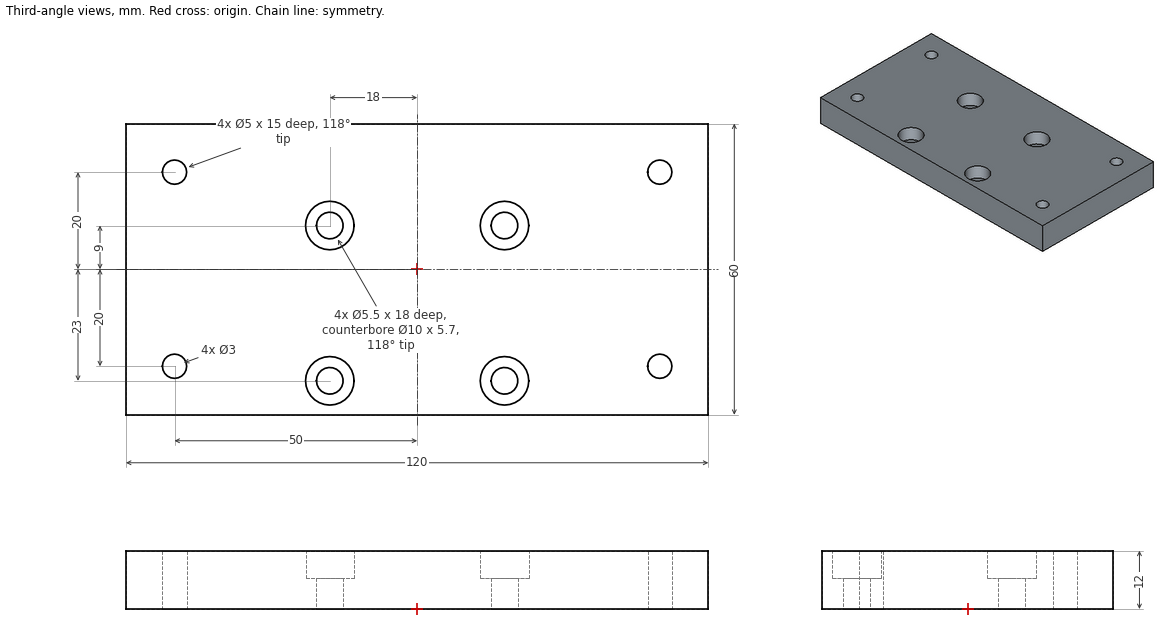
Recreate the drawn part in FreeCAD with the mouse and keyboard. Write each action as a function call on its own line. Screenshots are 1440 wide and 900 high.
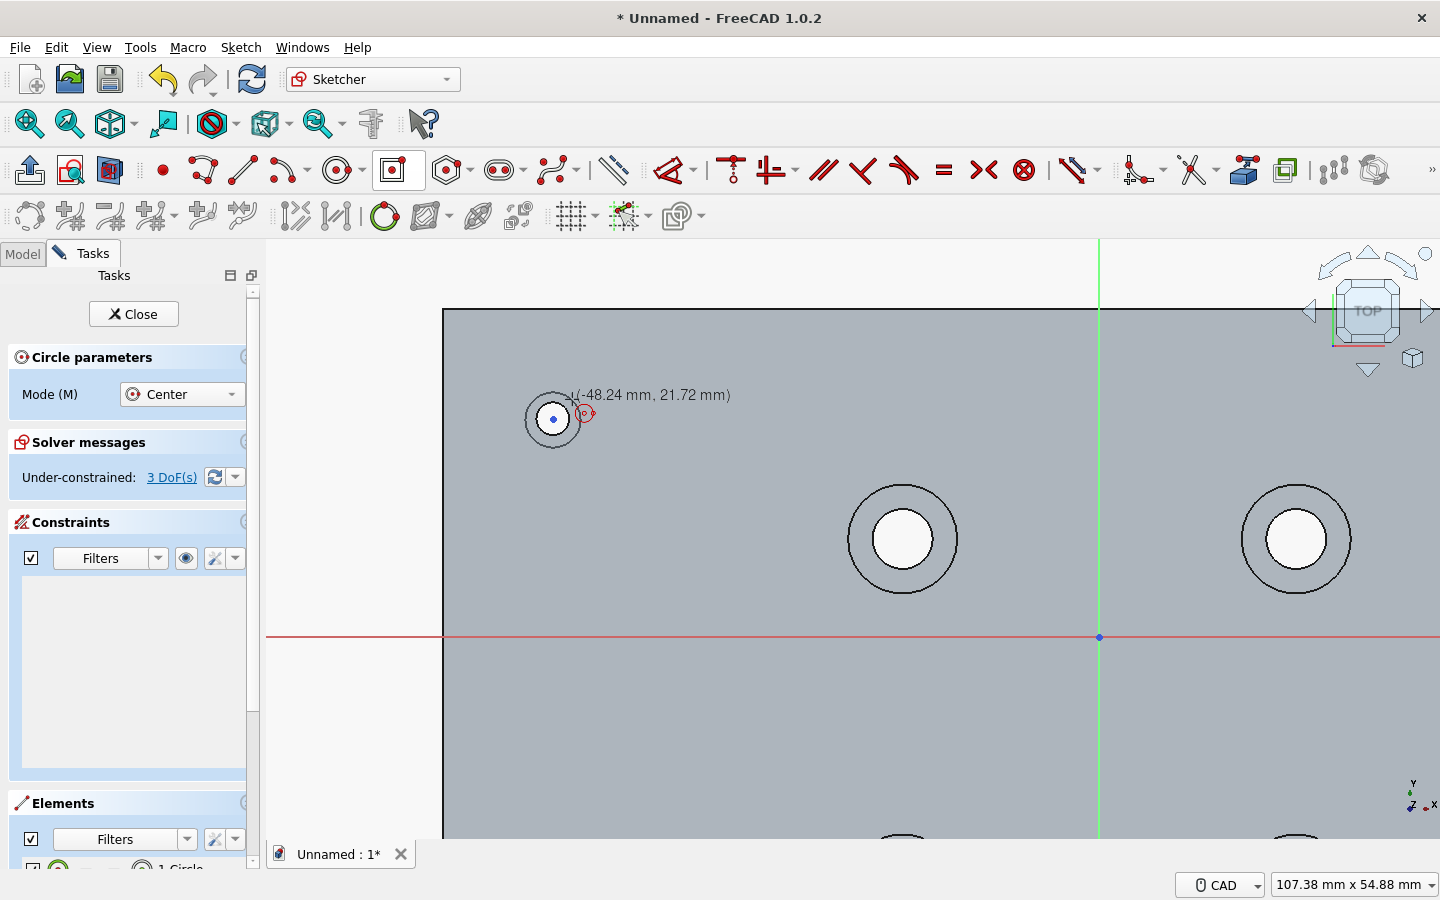
scroll(401, 419, down, 3)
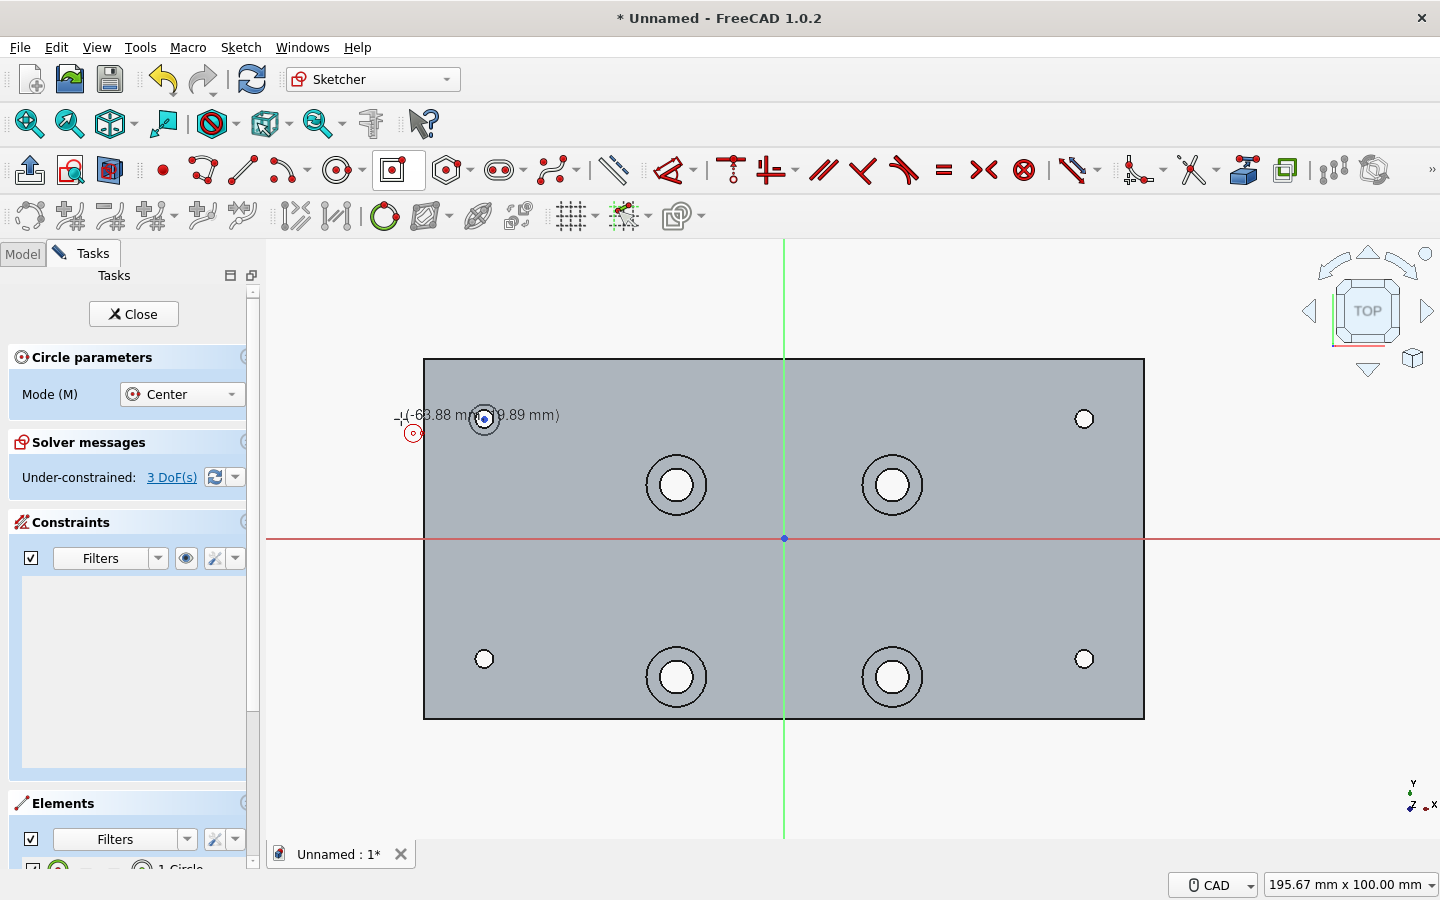
scroll(484, 659, up, 3)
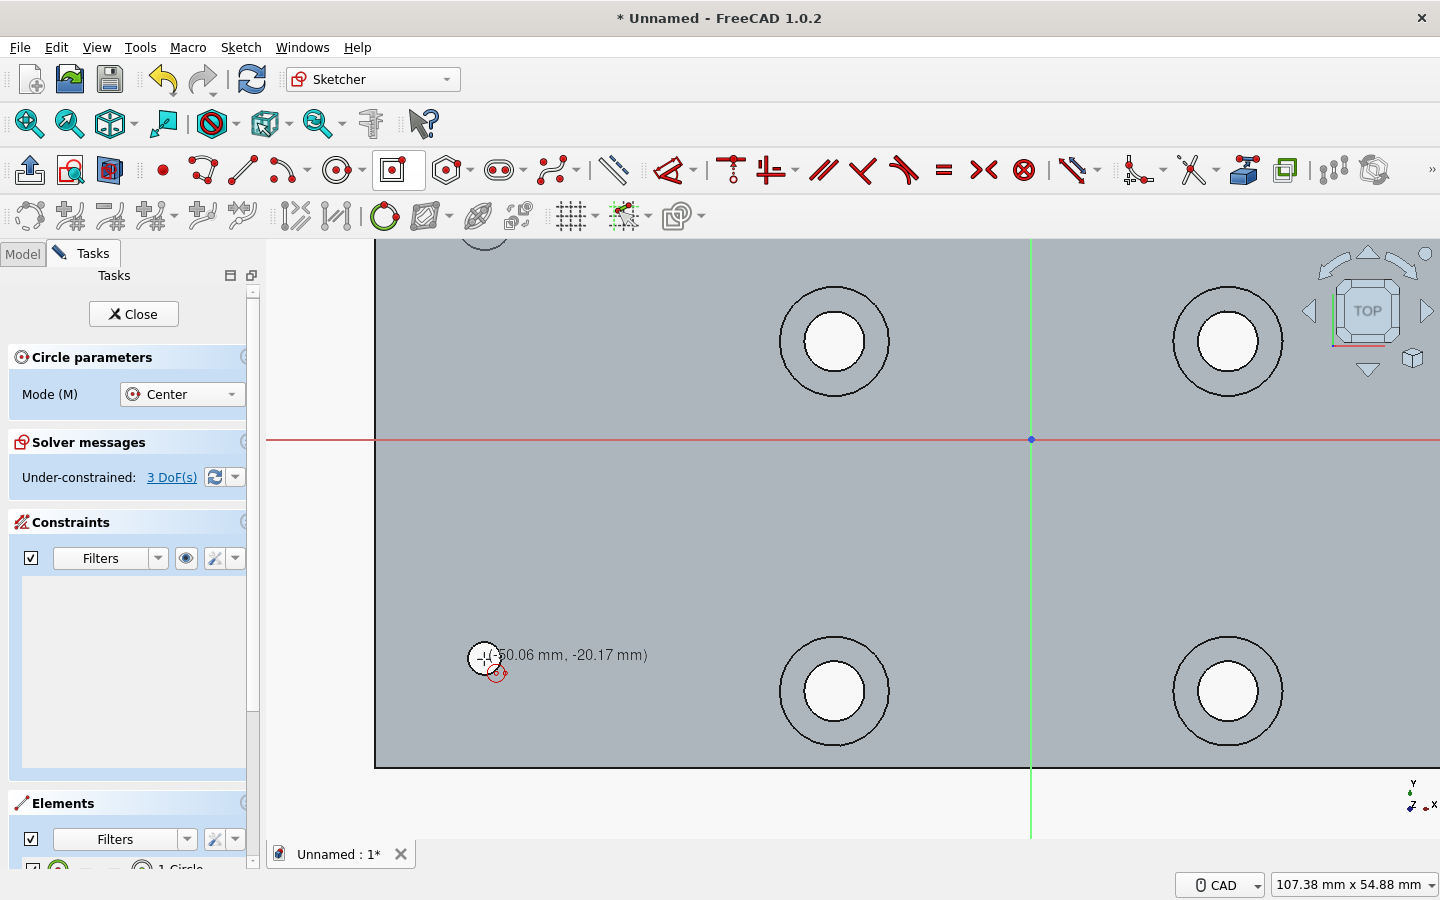
click(485, 658)
click(504, 639)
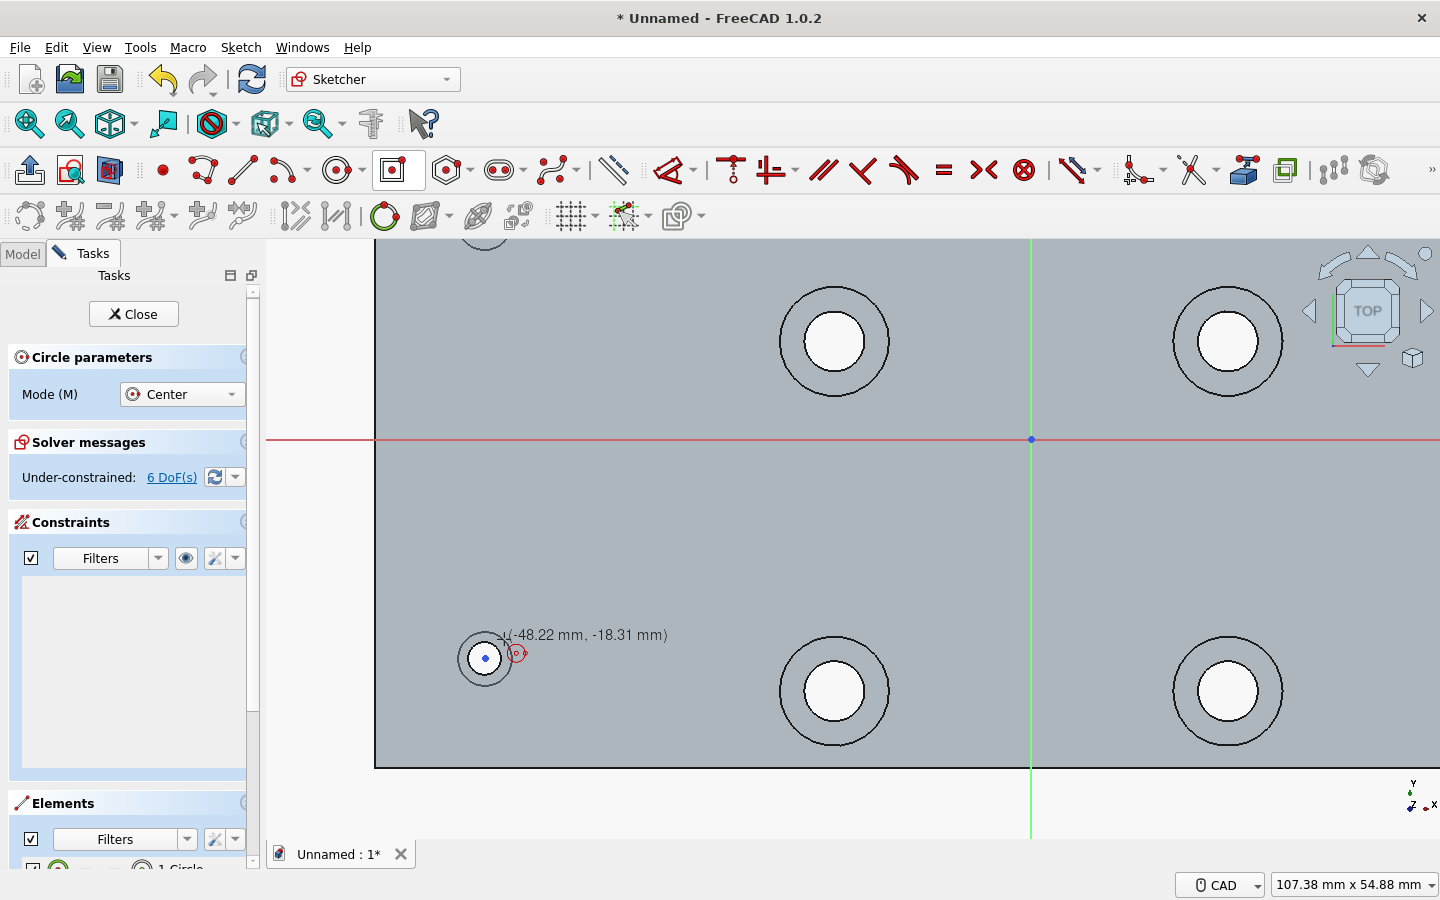
scroll(484, 660, down, 3)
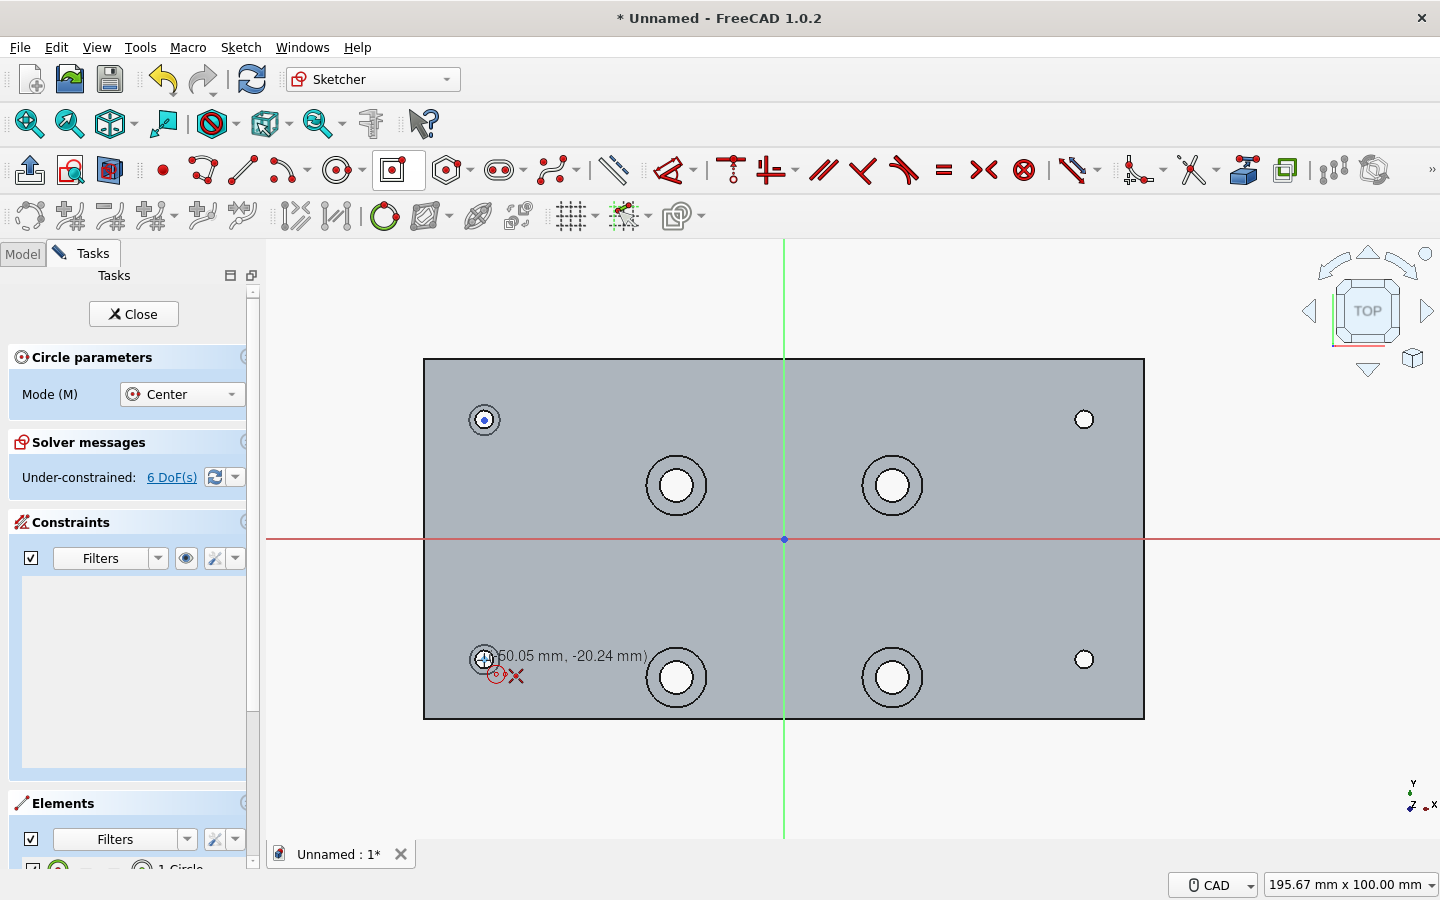
scroll(1084, 659, up, 3)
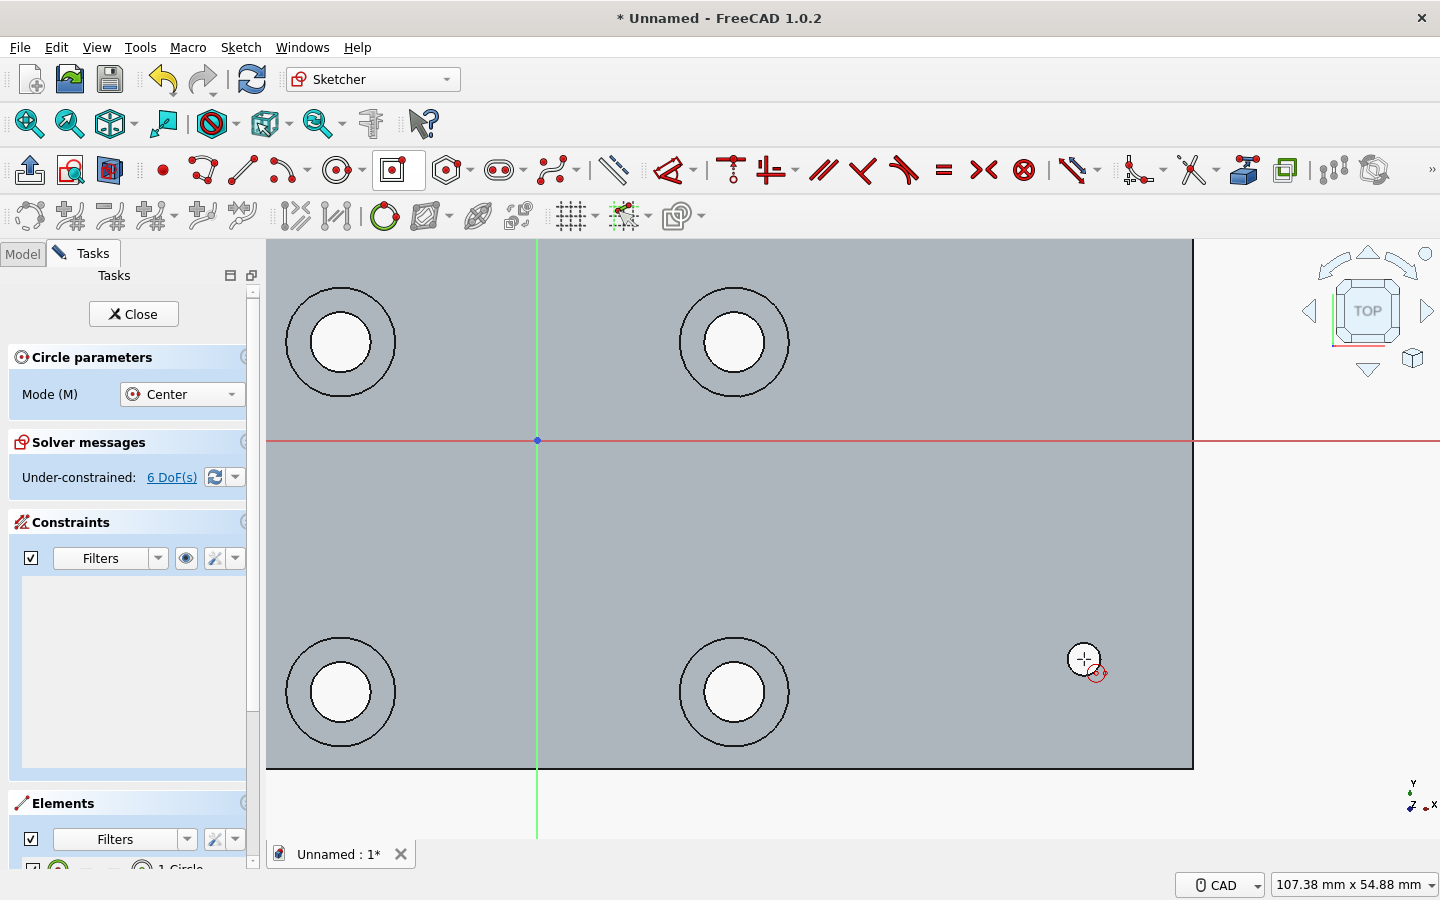
click(1084, 659)
click(1103, 640)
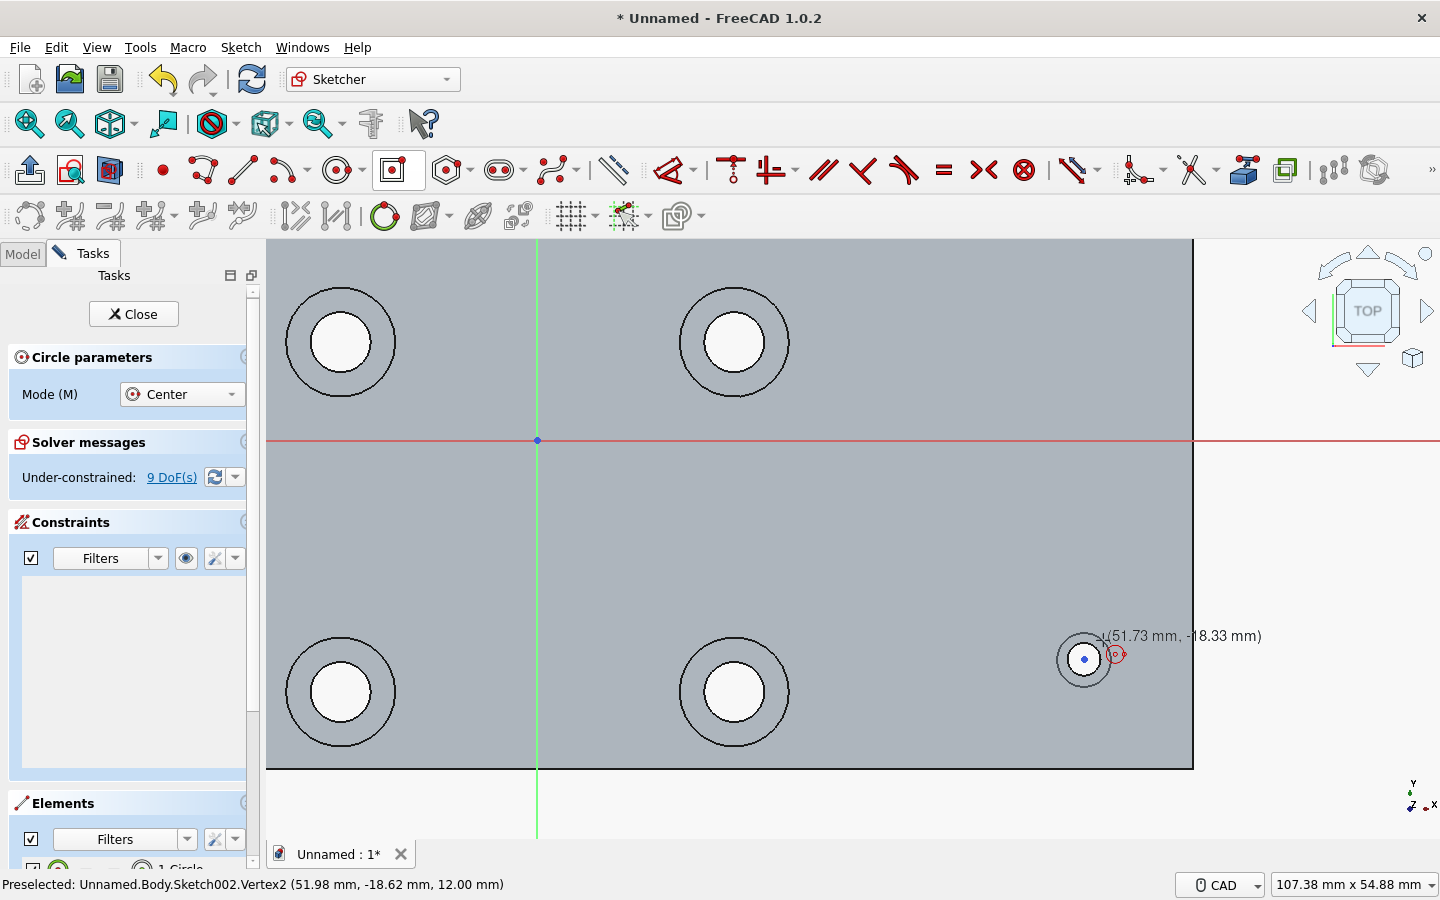
scroll(1085, 659, down, 3)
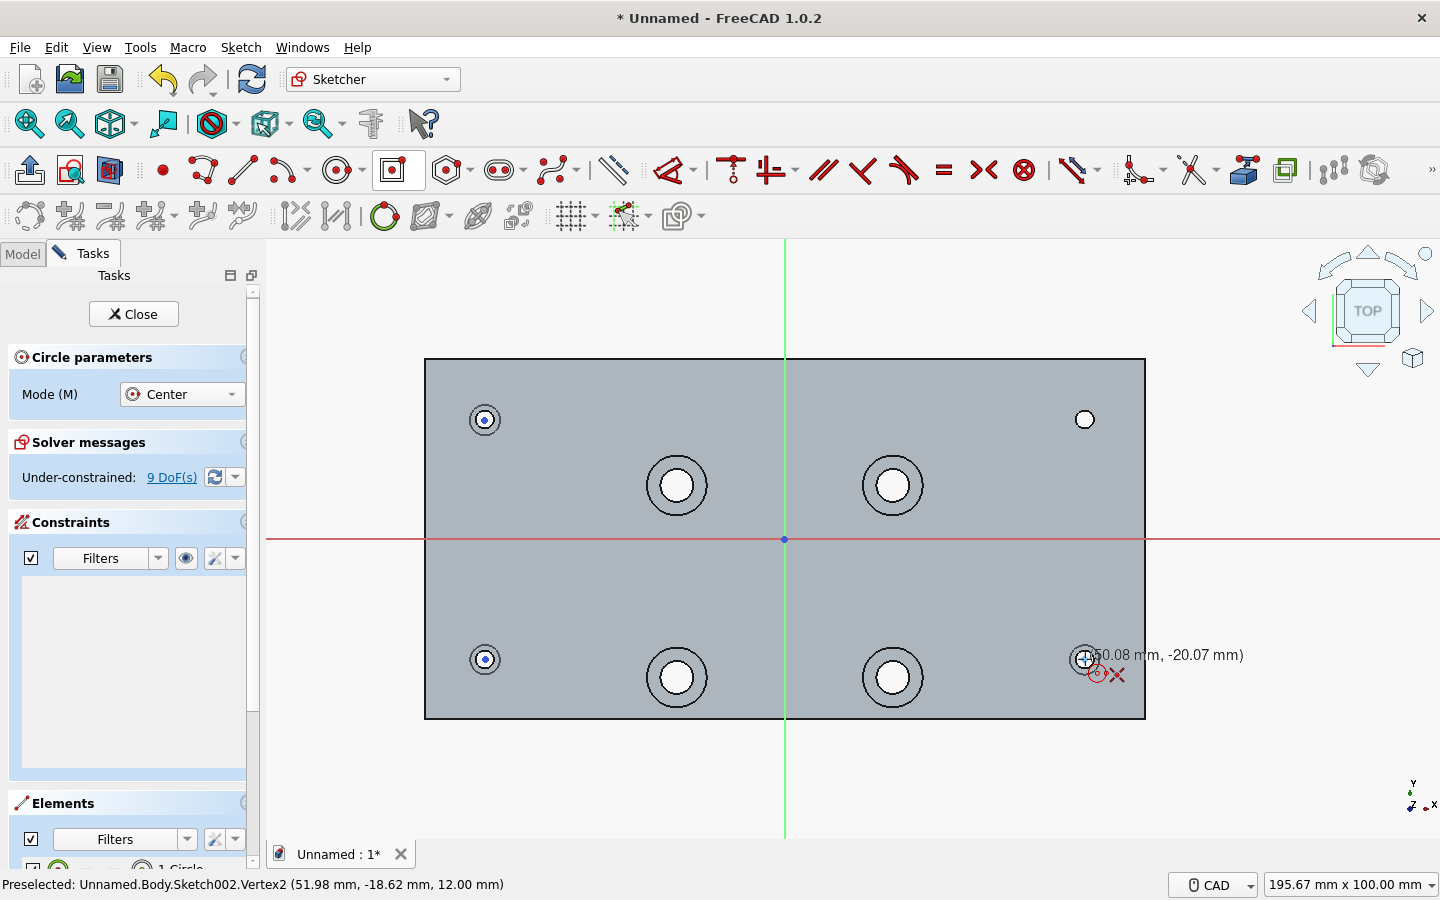
scroll(1085, 419, up, 3)